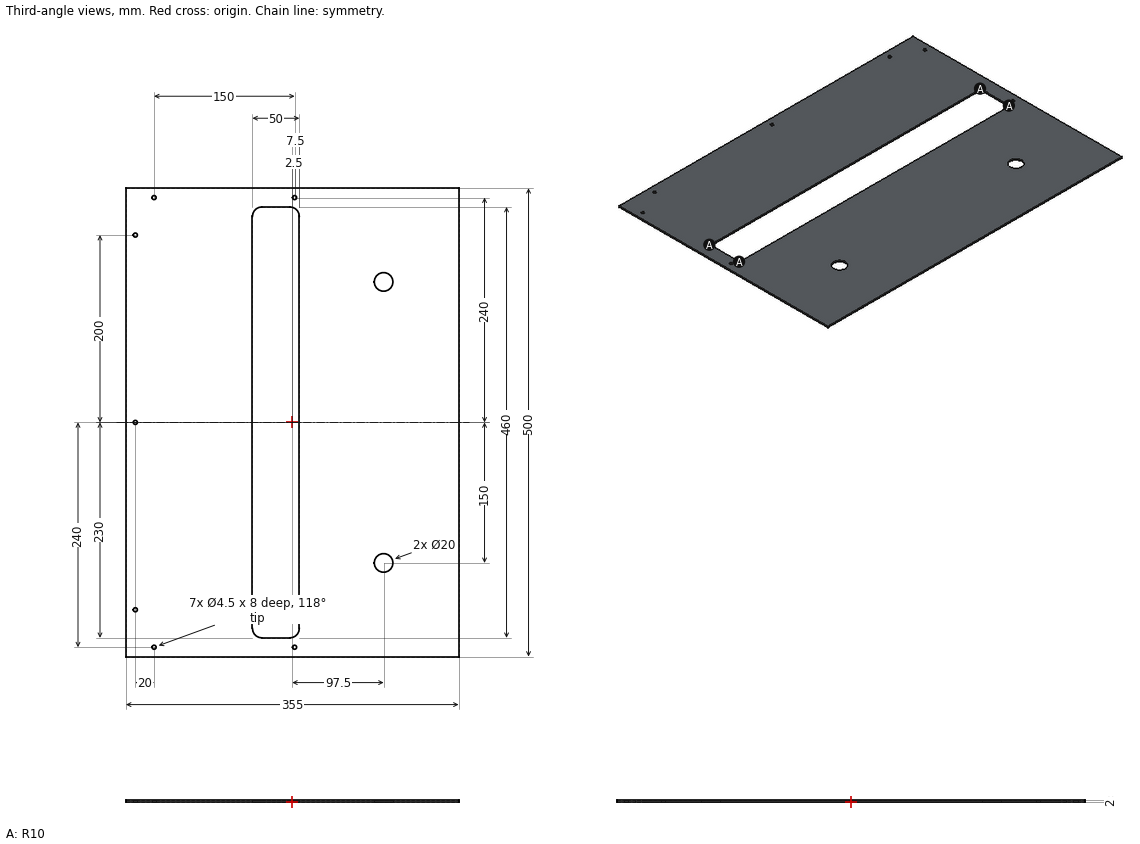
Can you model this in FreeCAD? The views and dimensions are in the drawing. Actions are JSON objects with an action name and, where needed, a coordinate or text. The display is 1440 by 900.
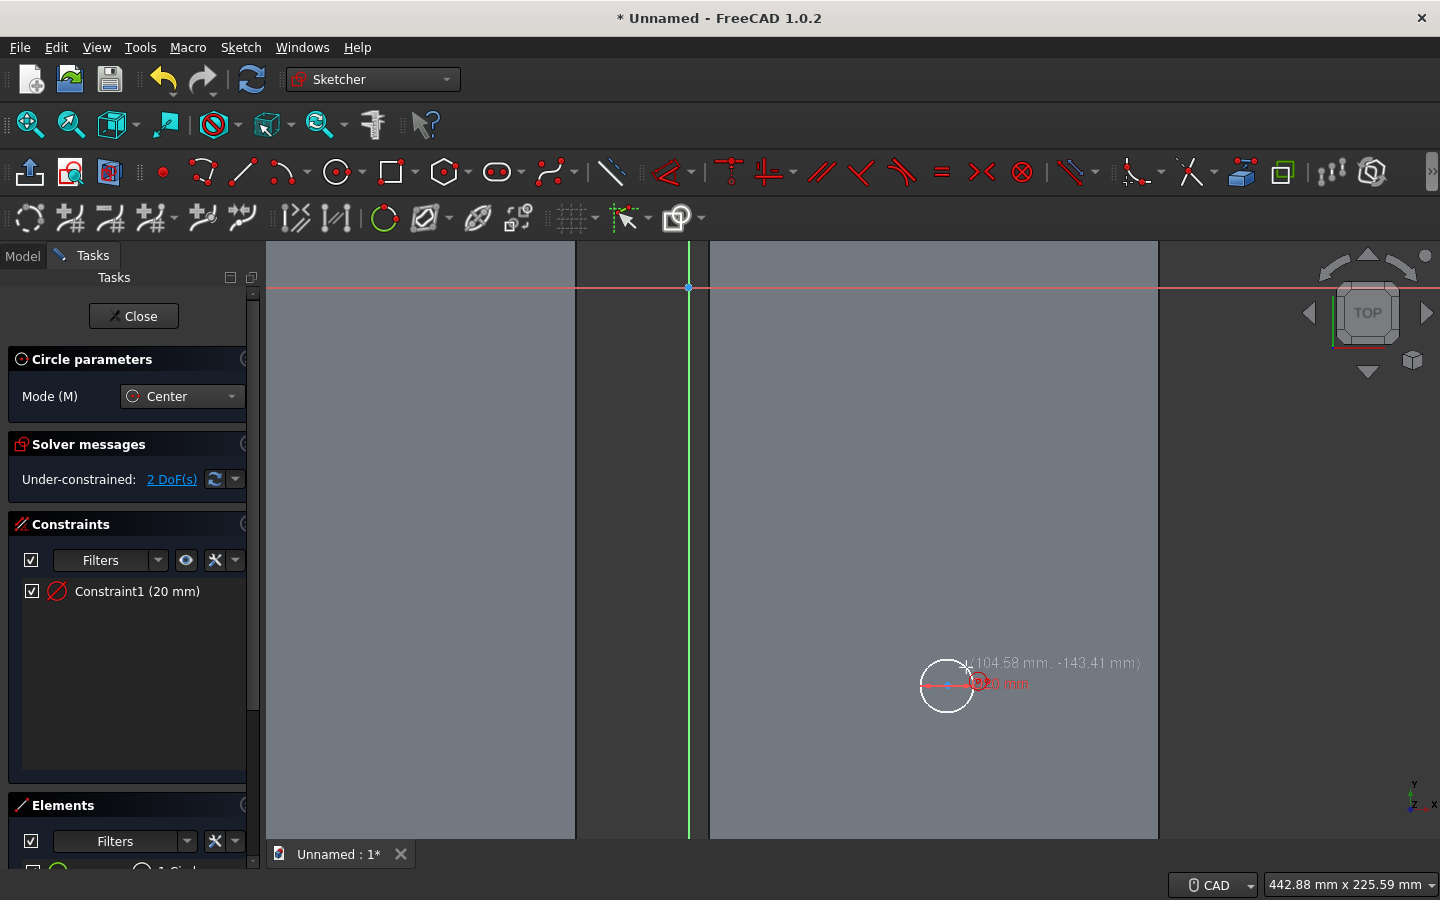
{"action": "scroll", "coordinate": [746, 746], "scroll_direction": "down", "scroll_amount": 4}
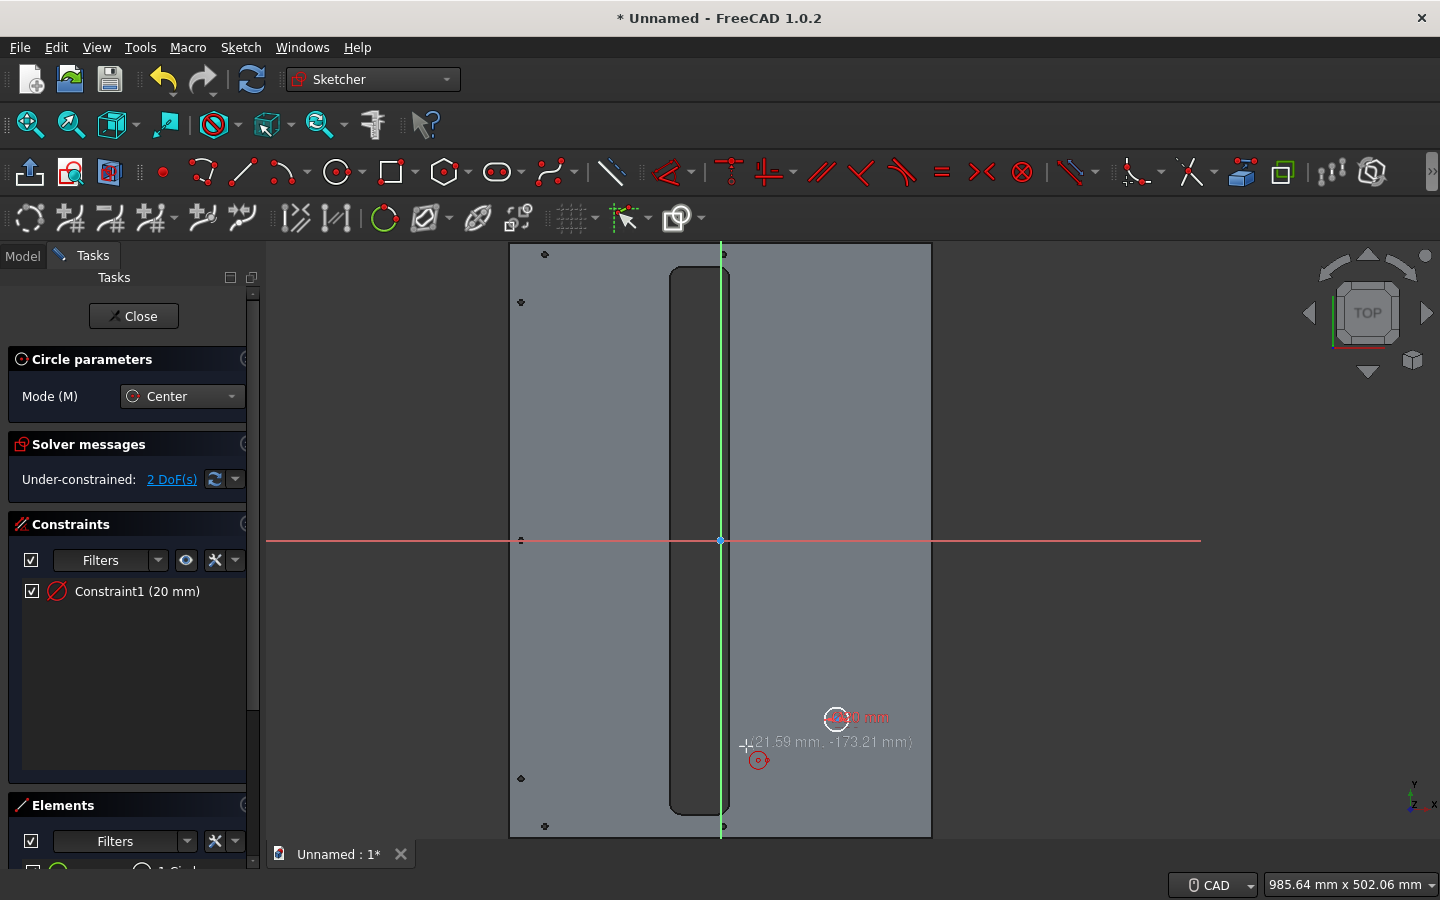
{"action": "scroll", "coordinate": [837, 362], "scroll_direction": "up", "scroll_amount": 4}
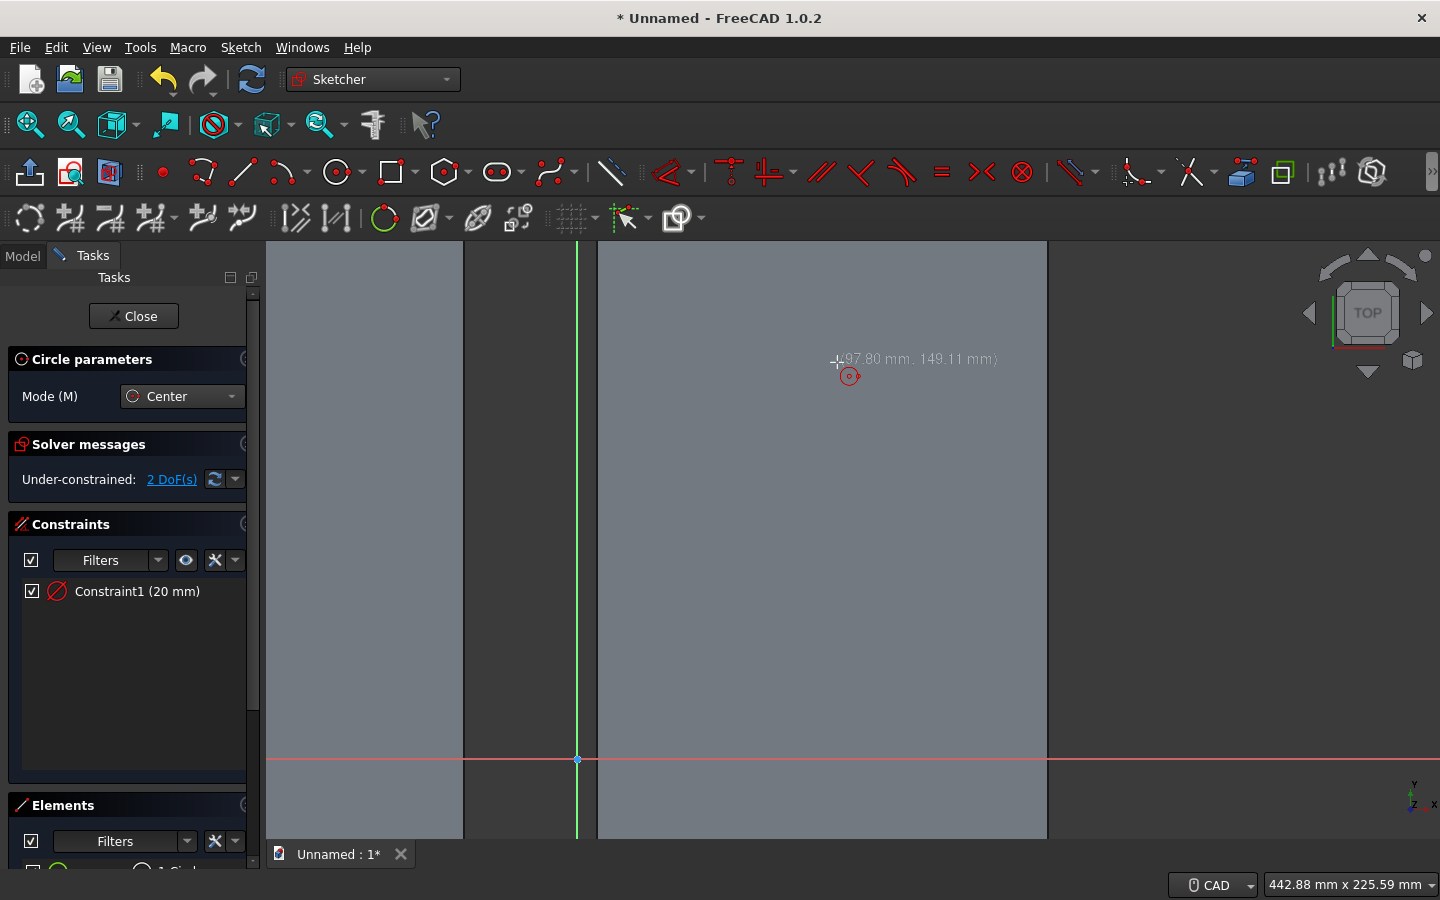
{"action": "left_click", "coordinate": [836, 362]}
{"action": "mouse_move", "coordinate": [854, 343]}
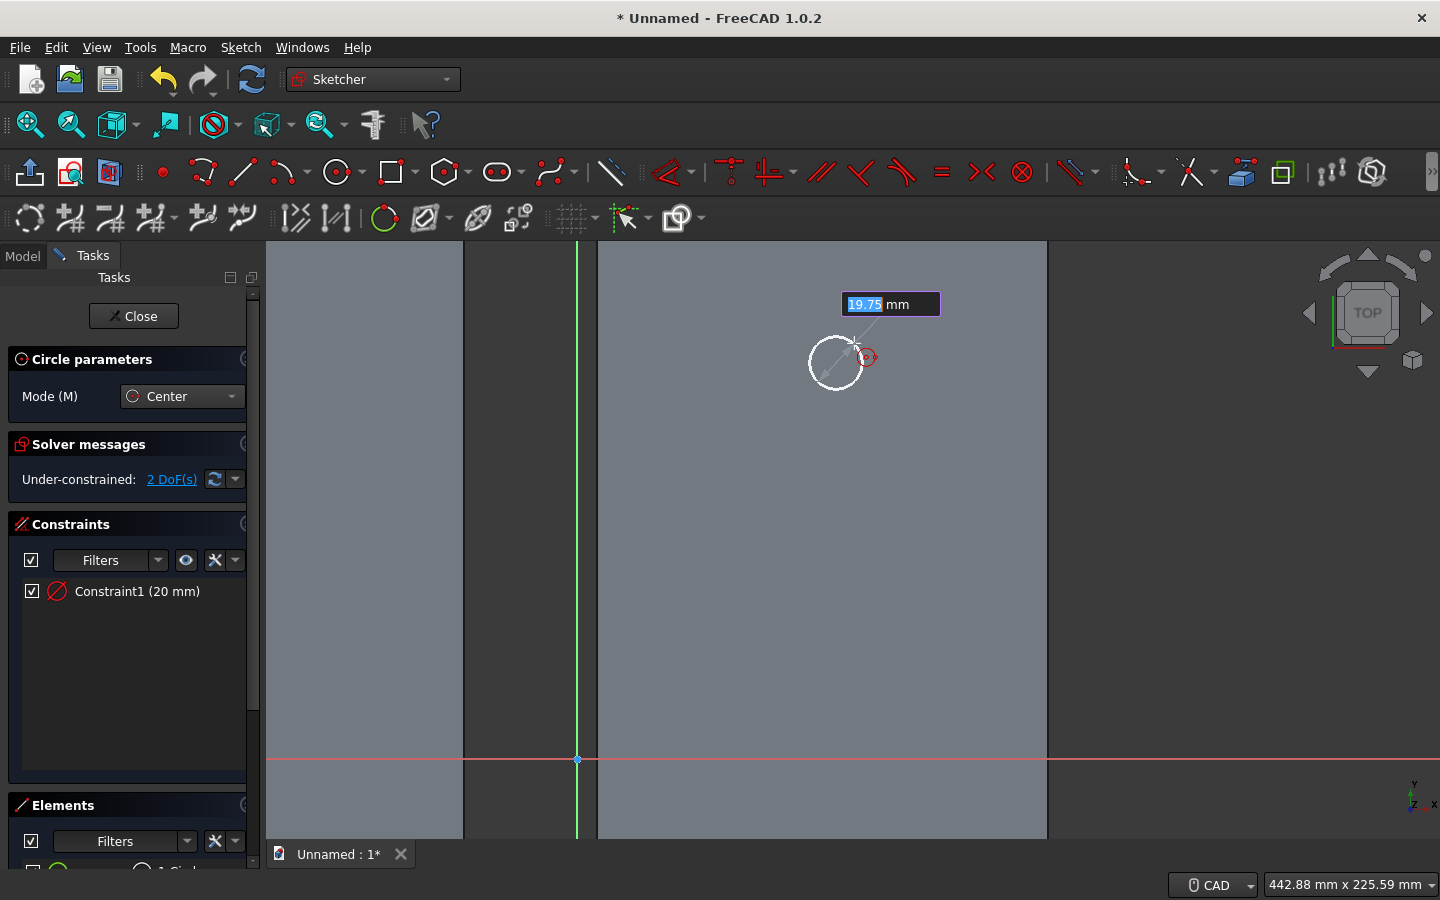
{"action": "type", "text": "20"}
{"action": "key", "text": "Return"}
{"action": "key", "text": "Escape"}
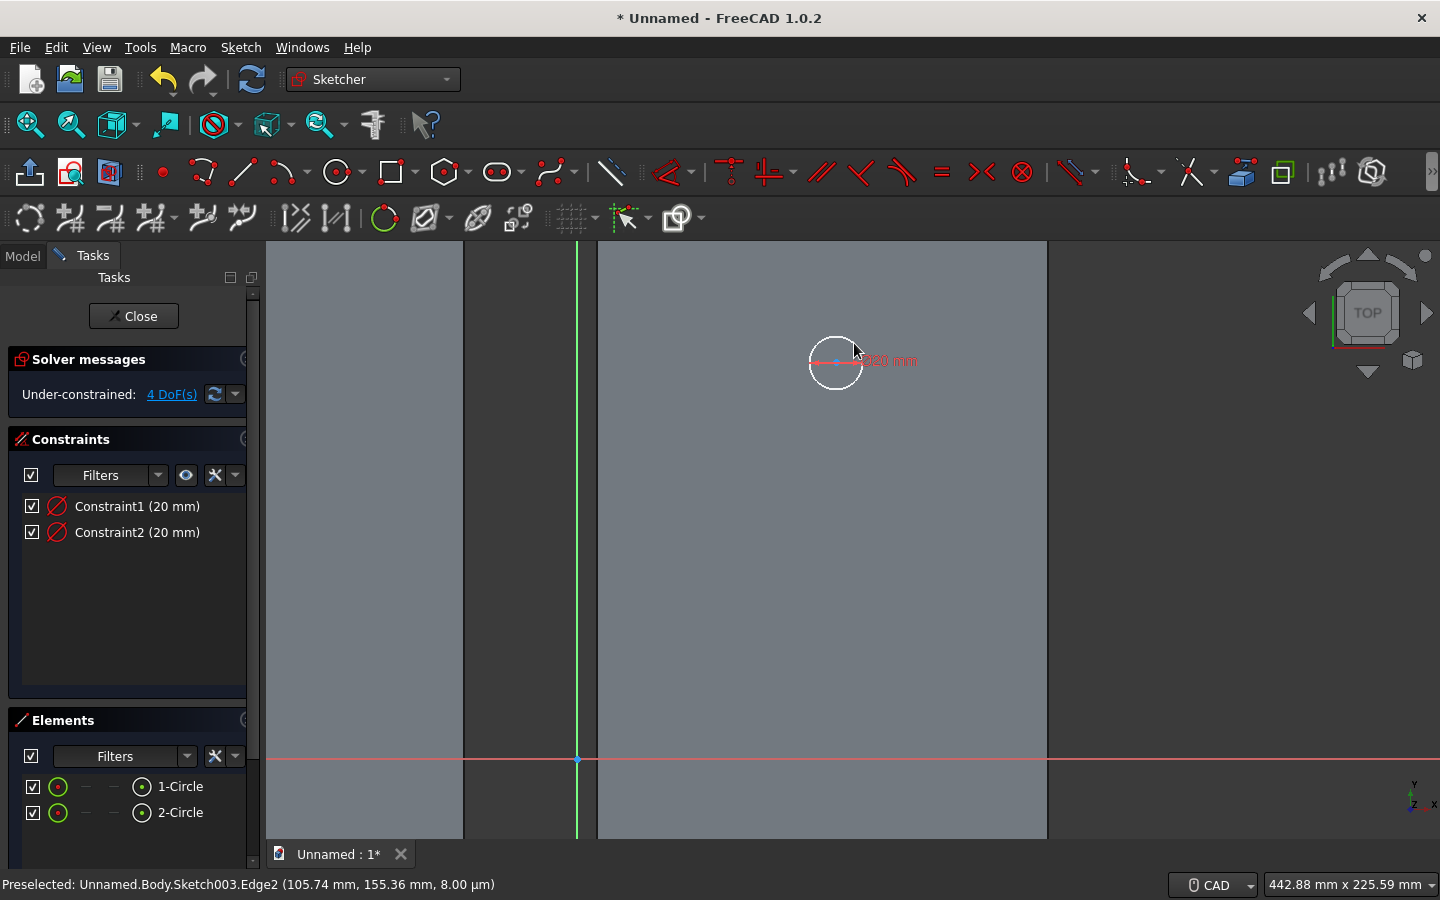
{"action": "scroll", "coordinate": [837, 361], "scroll_direction": "down", "scroll_amount": 4}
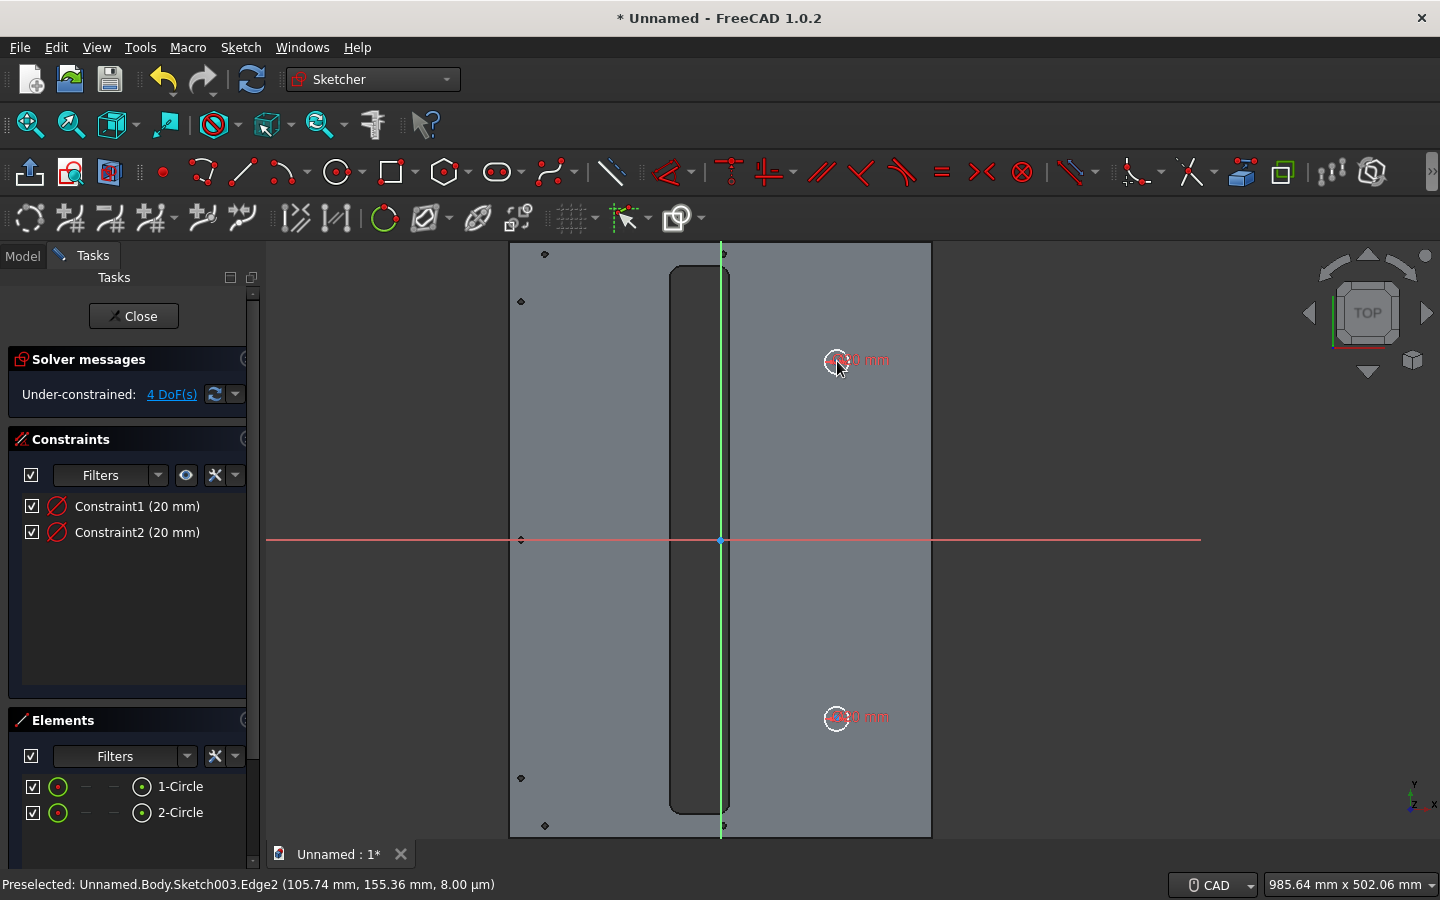
{"action": "left_click", "coordinate": [837, 719]}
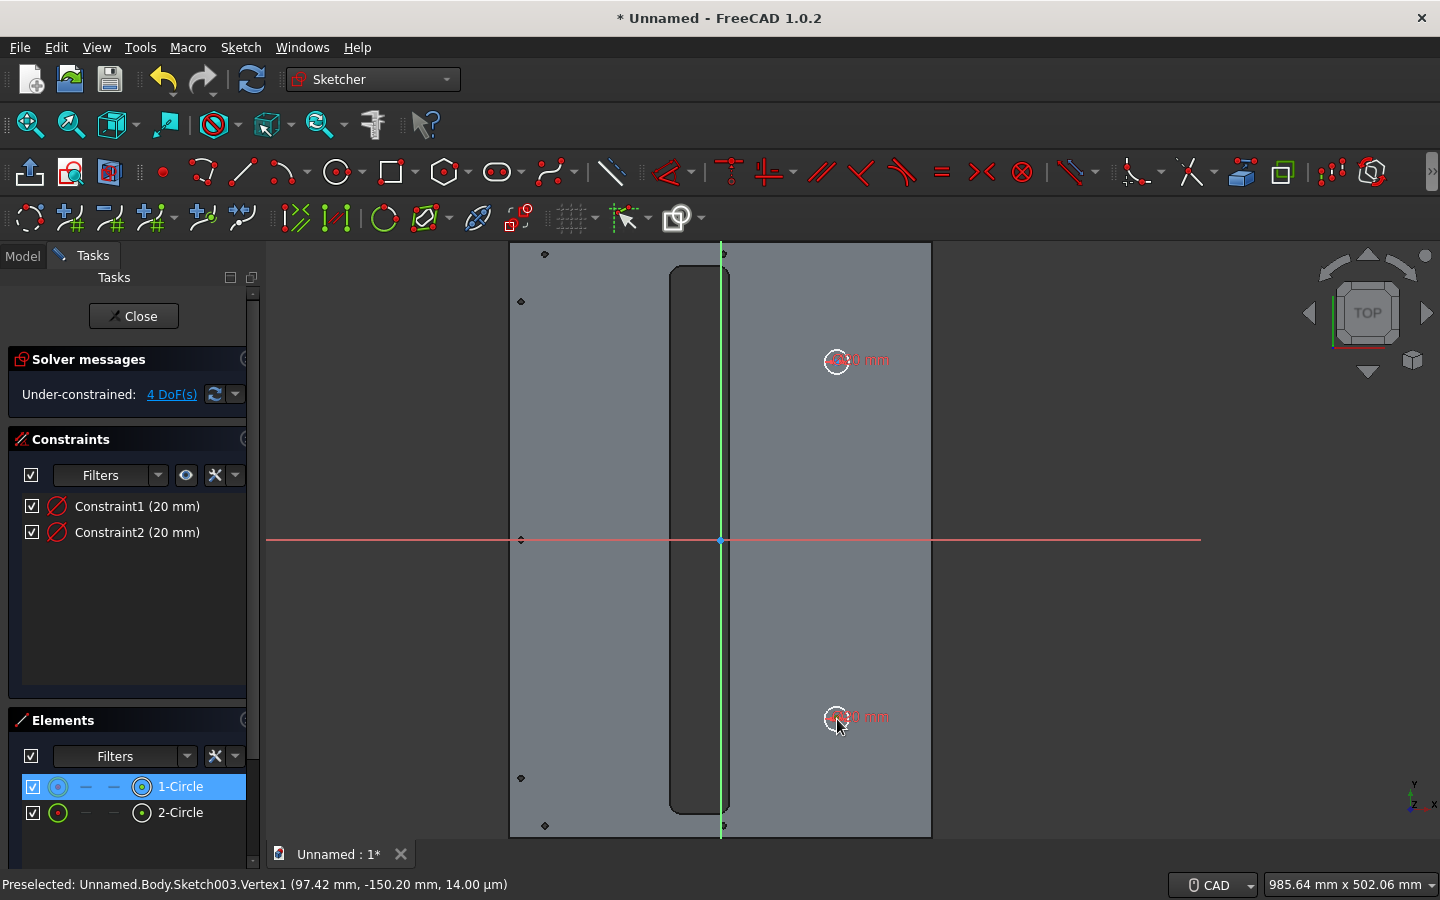
{"action": "left_click", "coordinate": [837, 362]}